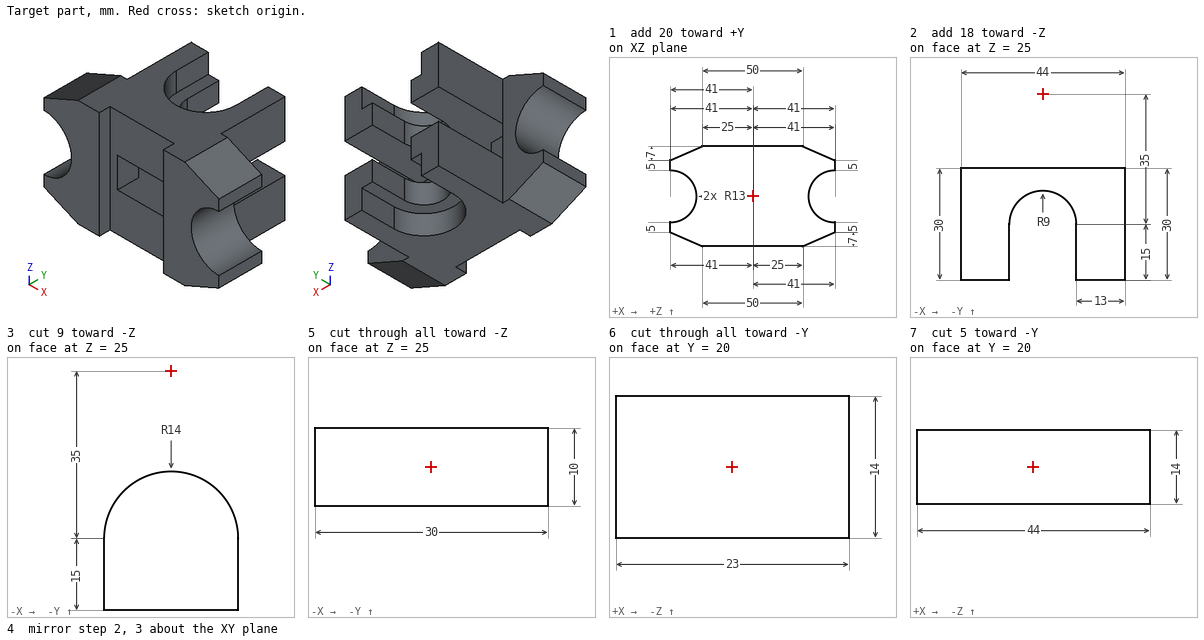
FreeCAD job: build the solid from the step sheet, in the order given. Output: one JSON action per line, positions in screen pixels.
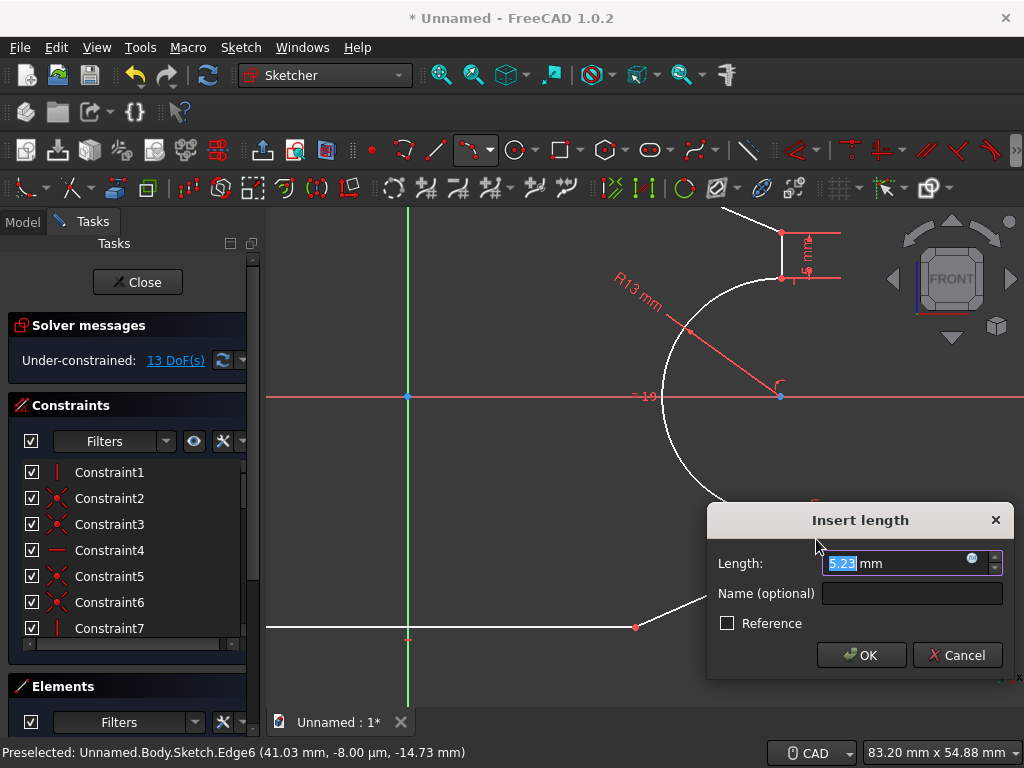
{"action": "type", "text": "5"}
{"action": "key", "text": "Return"}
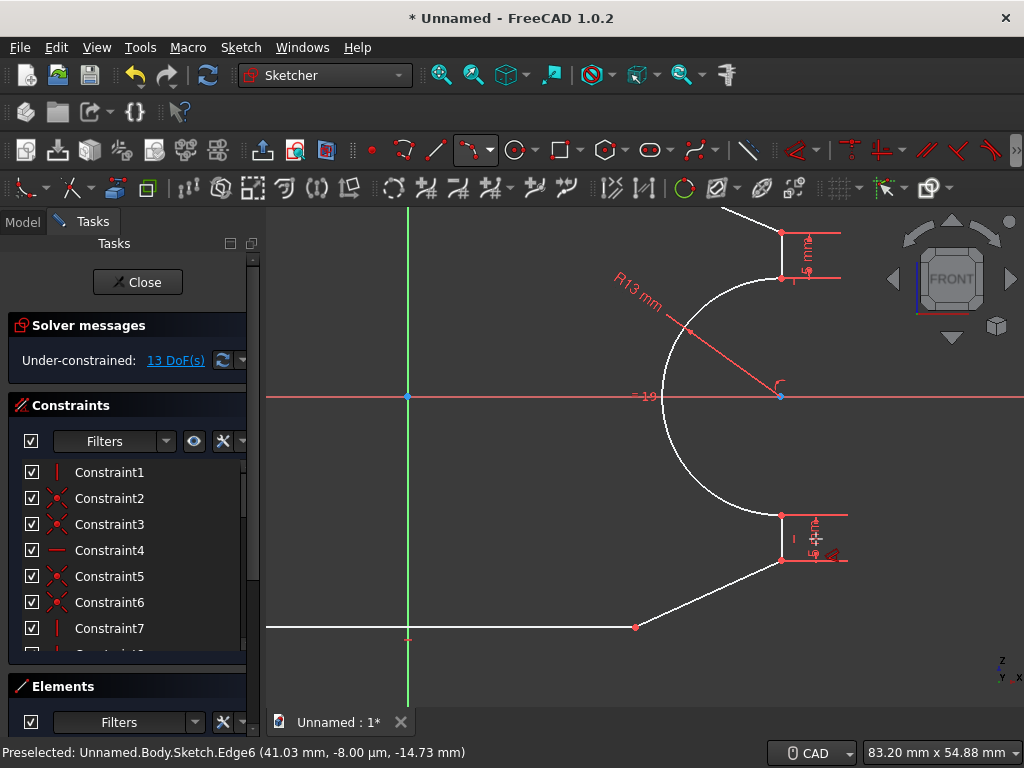
{"action": "scroll", "coordinate": [782, 530], "scroll_direction": "down", "scroll_amount": 3}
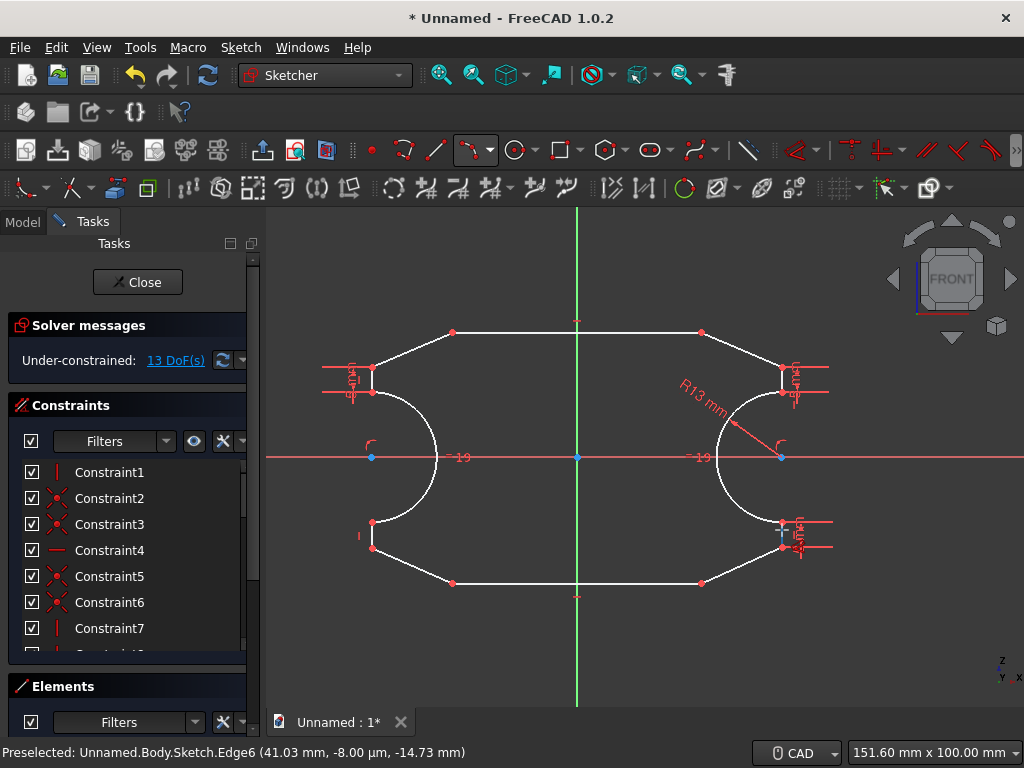
{"action": "scroll", "coordinate": [372, 540], "scroll_direction": "up", "scroll_amount": 3}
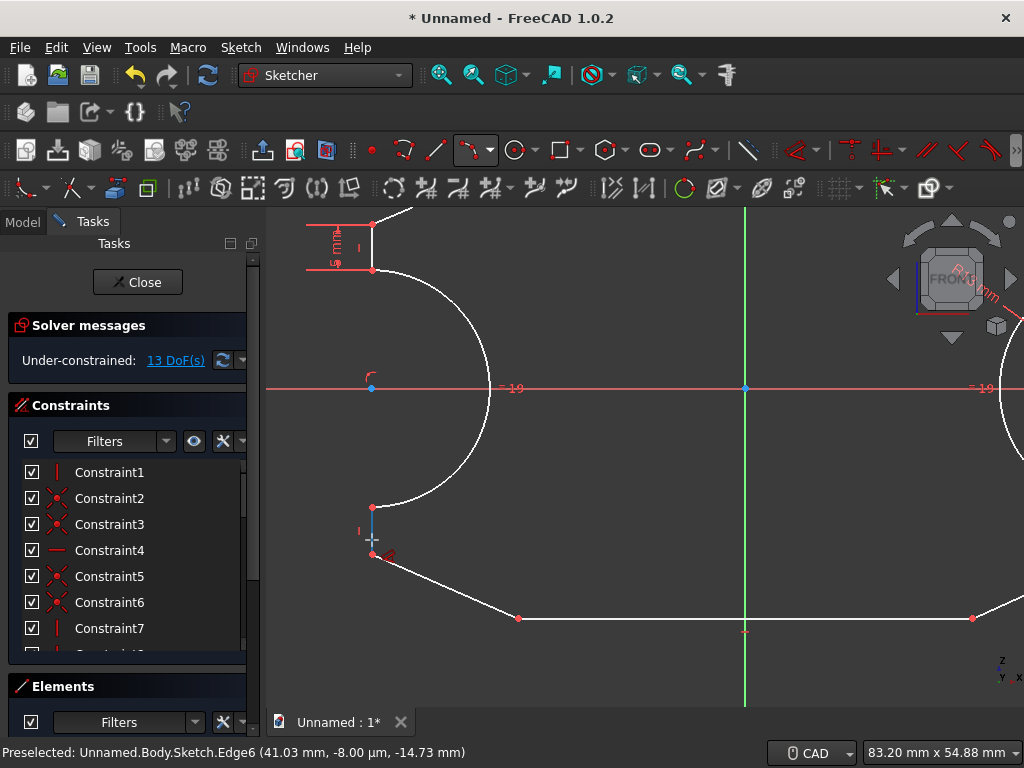
{"action": "left_click", "coordinate": [372, 540]}
{"action": "left_click", "coordinate": [338, 531]}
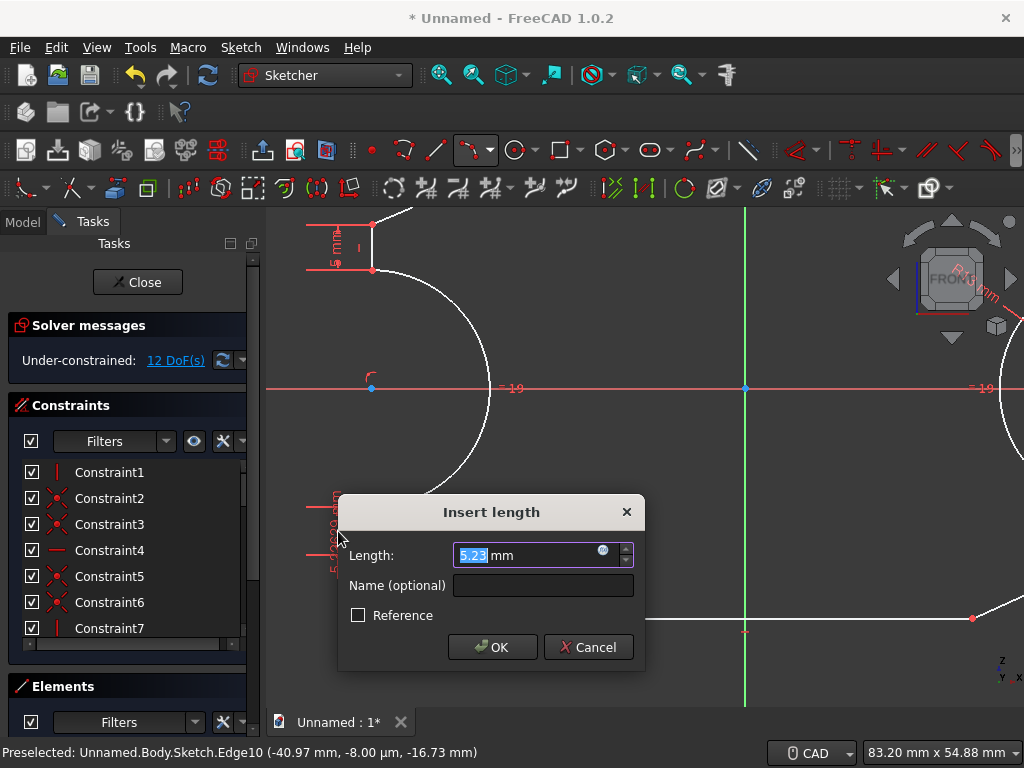
{"action": "type", "text": "5"}
{"action": "key", "text": "Return"}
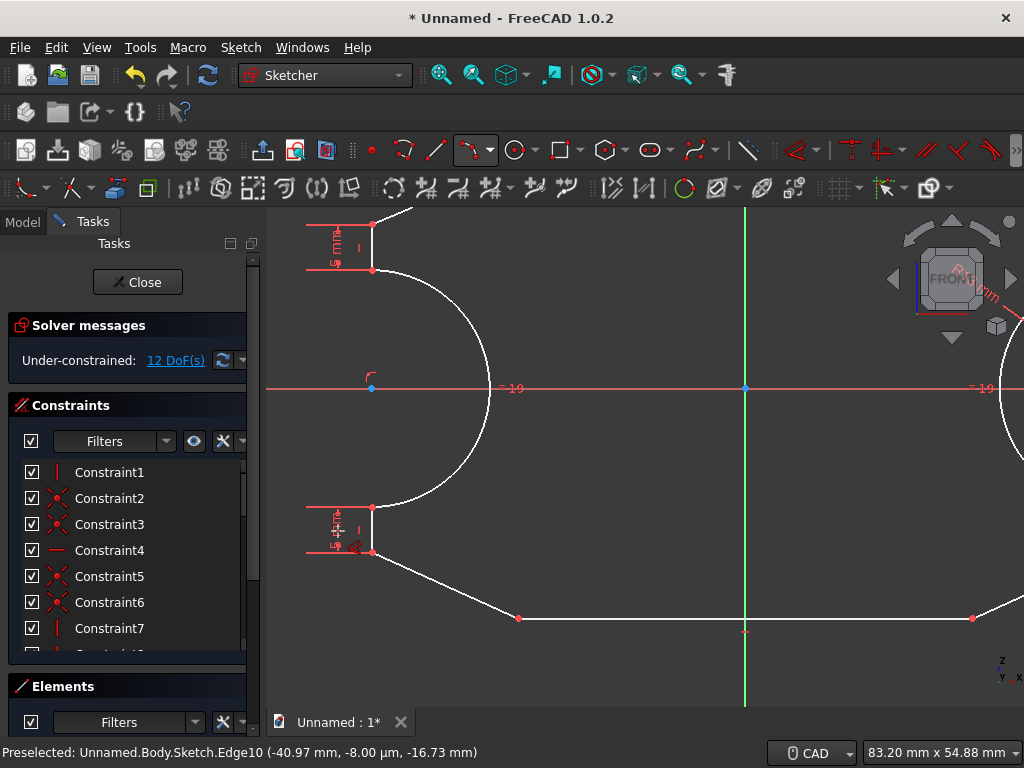
{"action": "scroll", "coordinate": [371, 540], "scroll_direction": "down", "scroll_amount": 3}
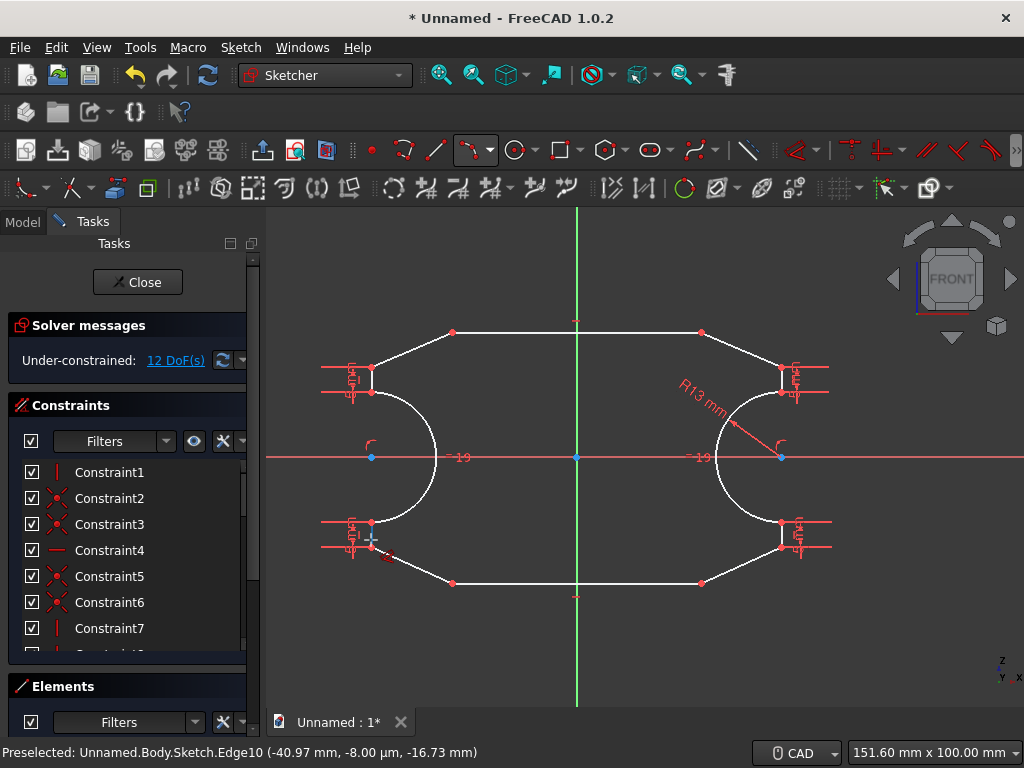
{"action": "left_click", "coordinate": [527, 333]}
{"action": "left_click", "coordinate": [519, 299]}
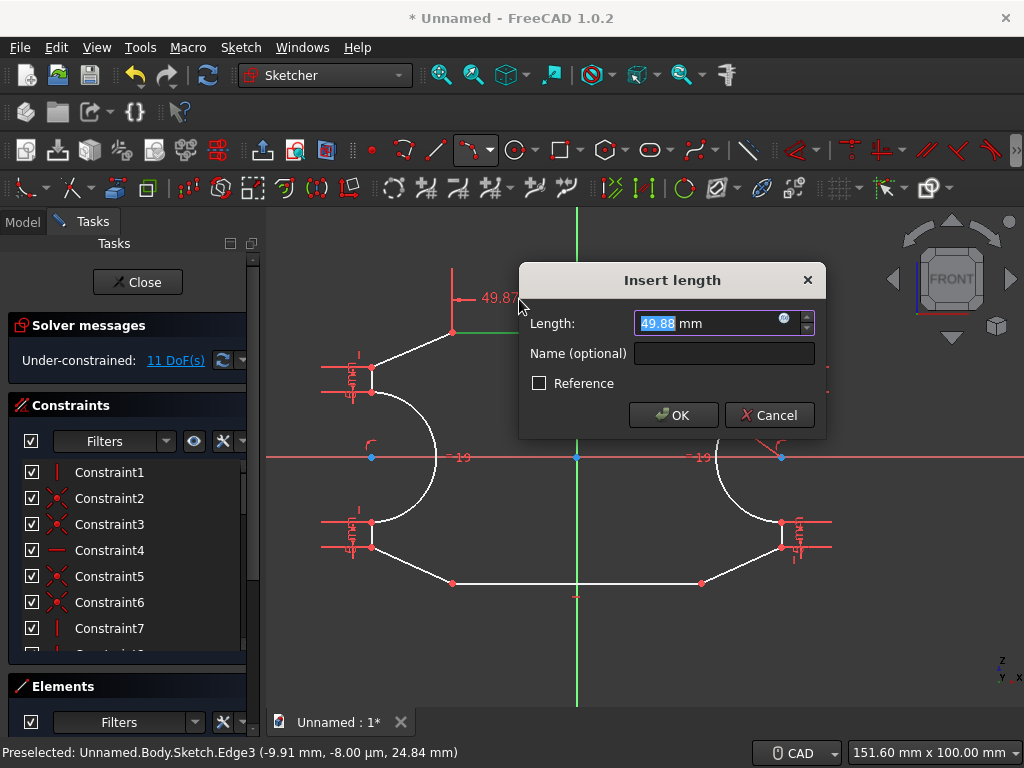
{"action": "type", "text": "50"}
{"action": "key", "text": "Return"}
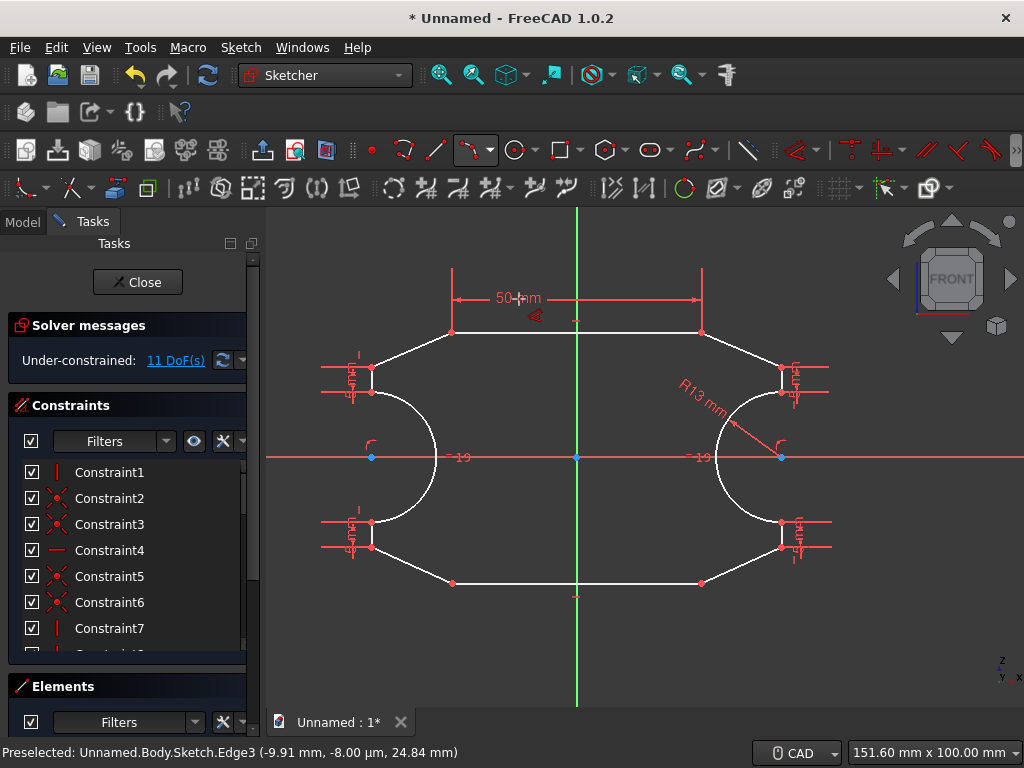
{"action": "left_click", "coordinate": [627, 584]}
{"action": "left_click", "coordinate": [519, 618]}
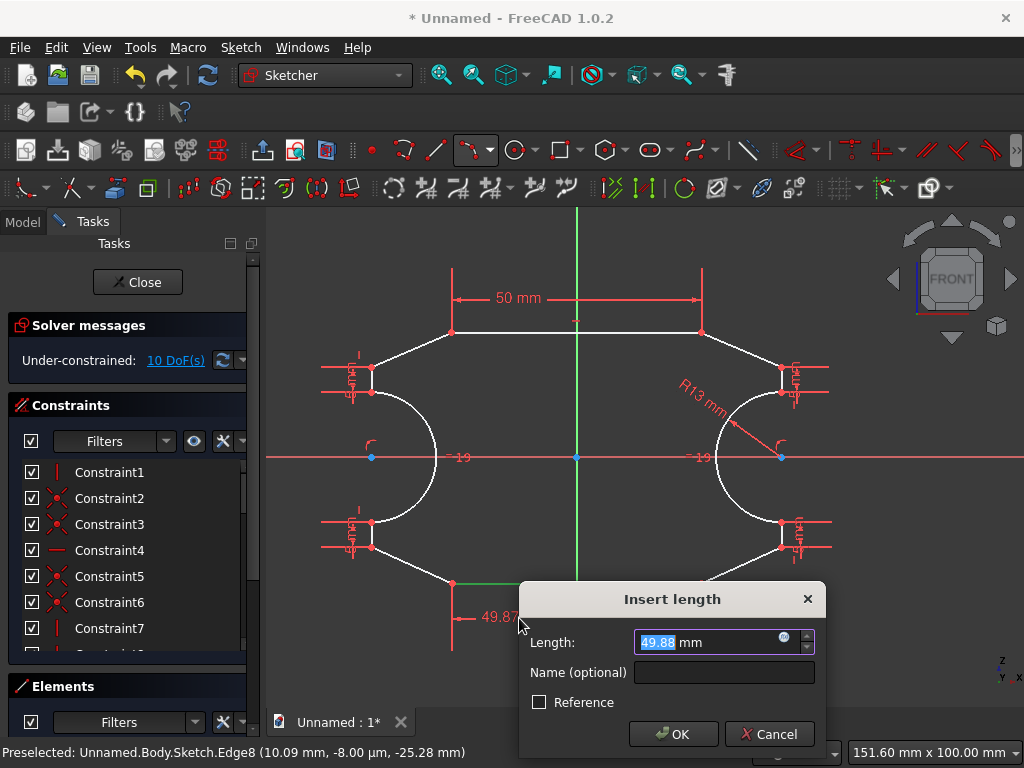
{"action": "type", "text": "50"}
{"action": "key", "text": "Return"}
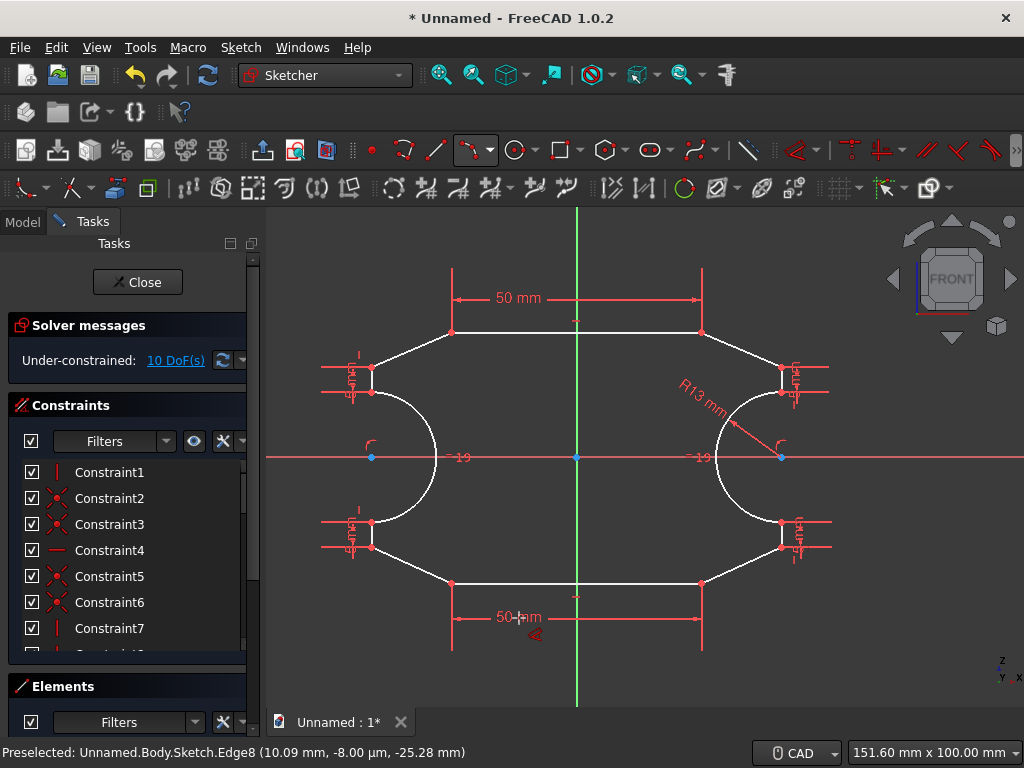
{"action": "left_click", "coordinate": [396, 357]}
{"action": "left_click", "coordinate": [338, 350]}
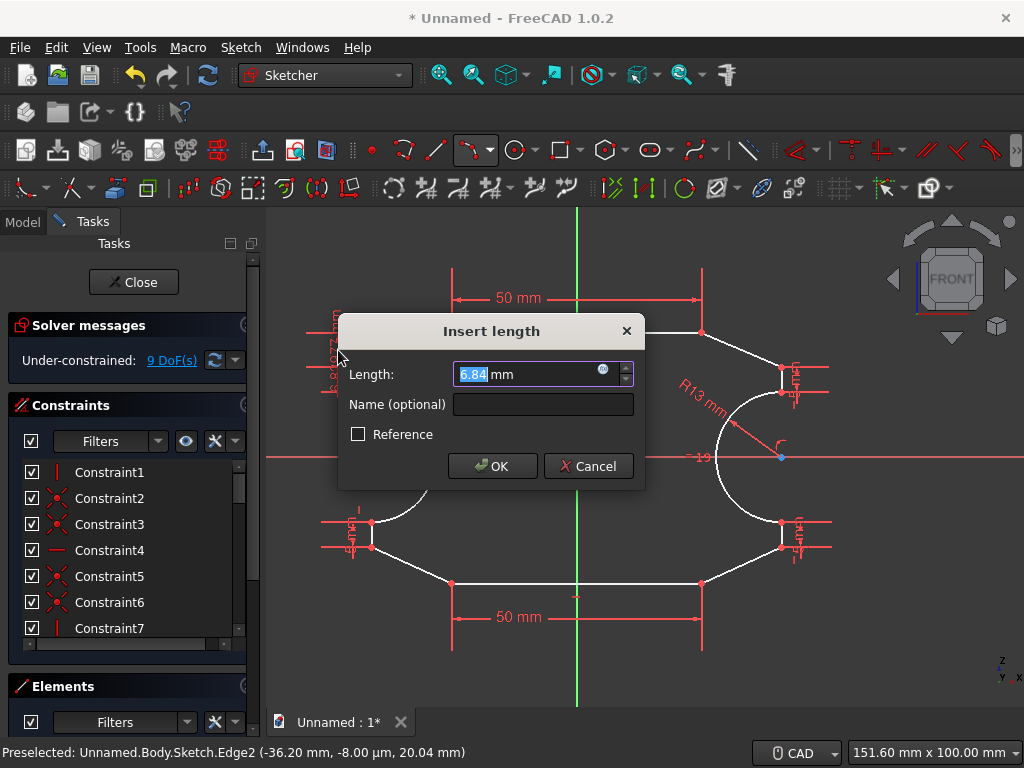
{"action": "type", "text": "7"}
{"action": "key", "text": "Return"}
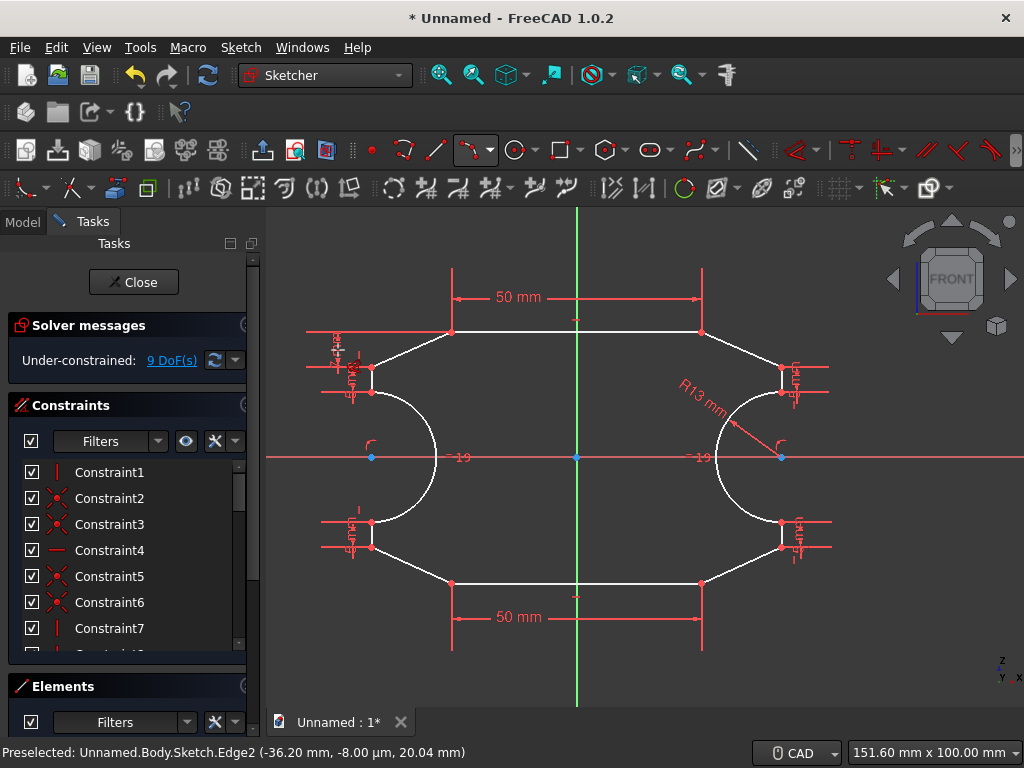
{"action": "left_click", "coordinate": [758, 558]}
{"action": "left_click", "coordinate": [816, 565]}